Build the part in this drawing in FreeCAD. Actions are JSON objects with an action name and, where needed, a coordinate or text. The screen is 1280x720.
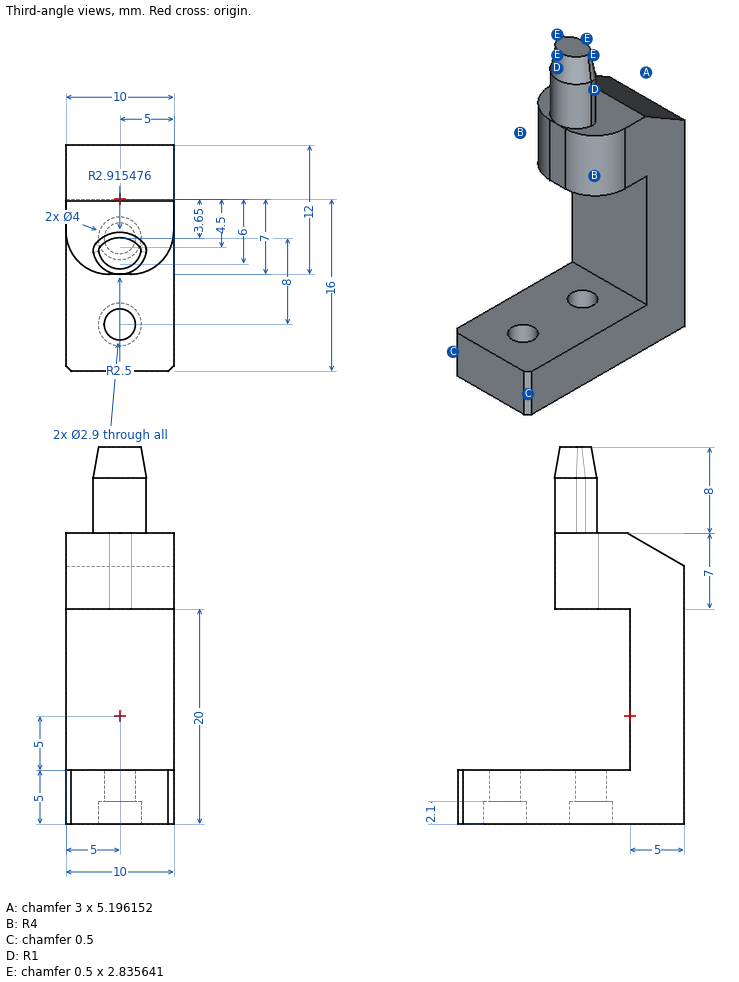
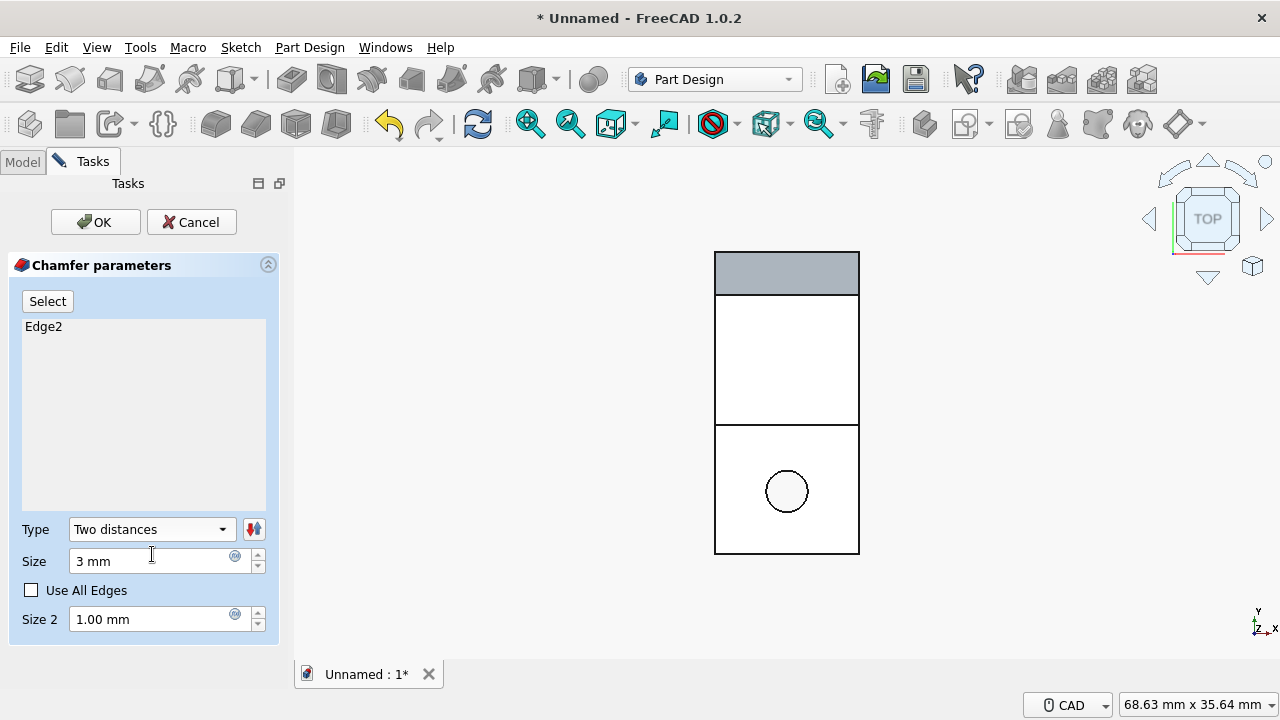
{"action": "triple_click", "coordinate": [160, 619]}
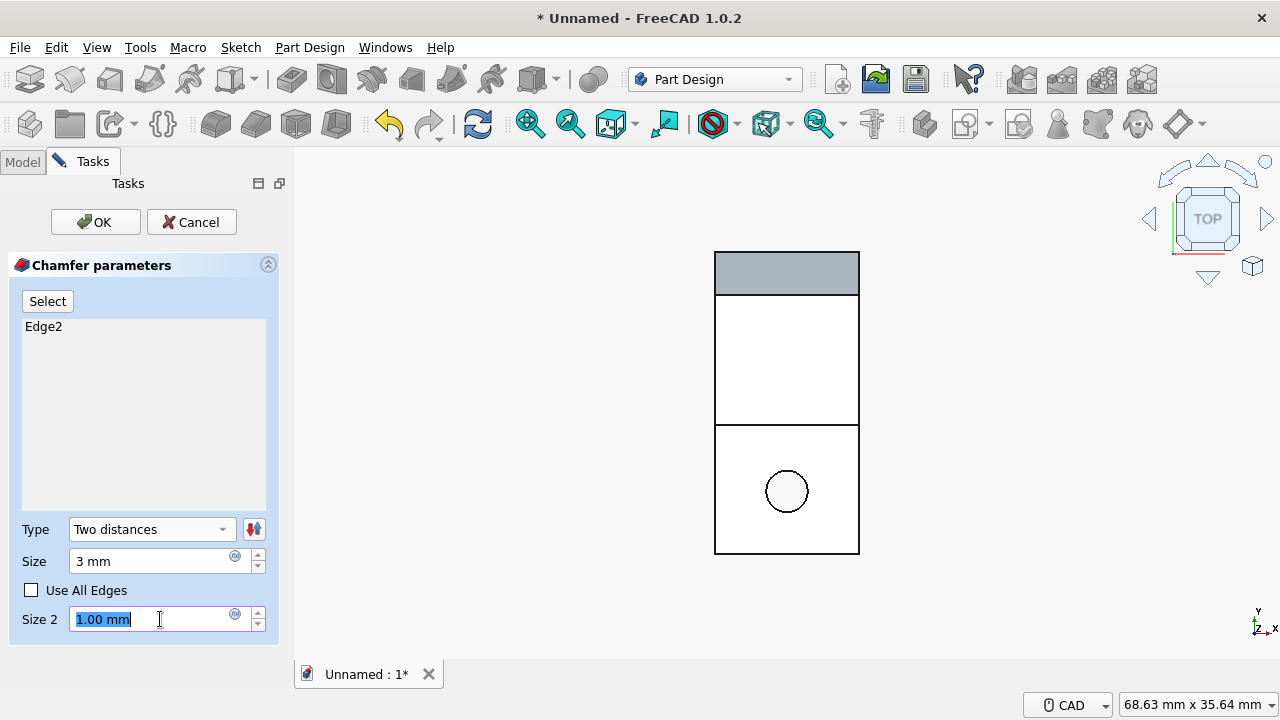
{"action": "type", "text": "5.196152"}
{"action": "key", "text": "Tab"}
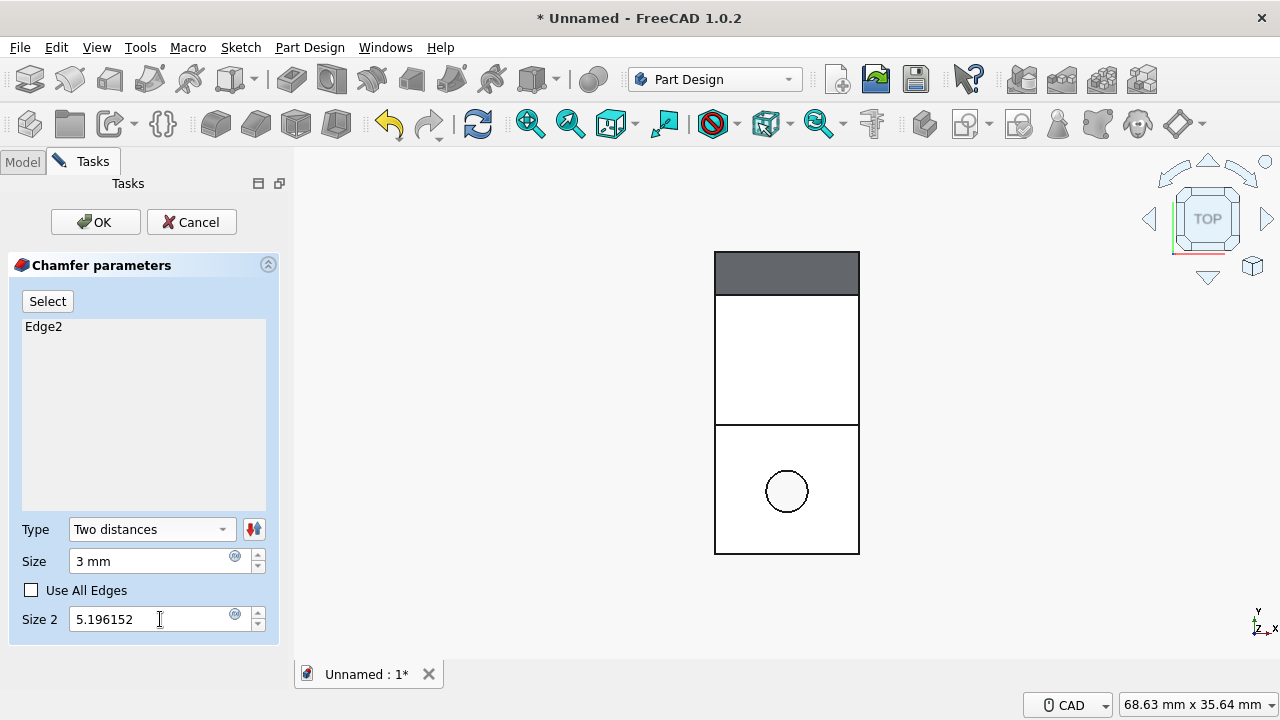
{"action": "left_click", "coordinate": [254, 530]}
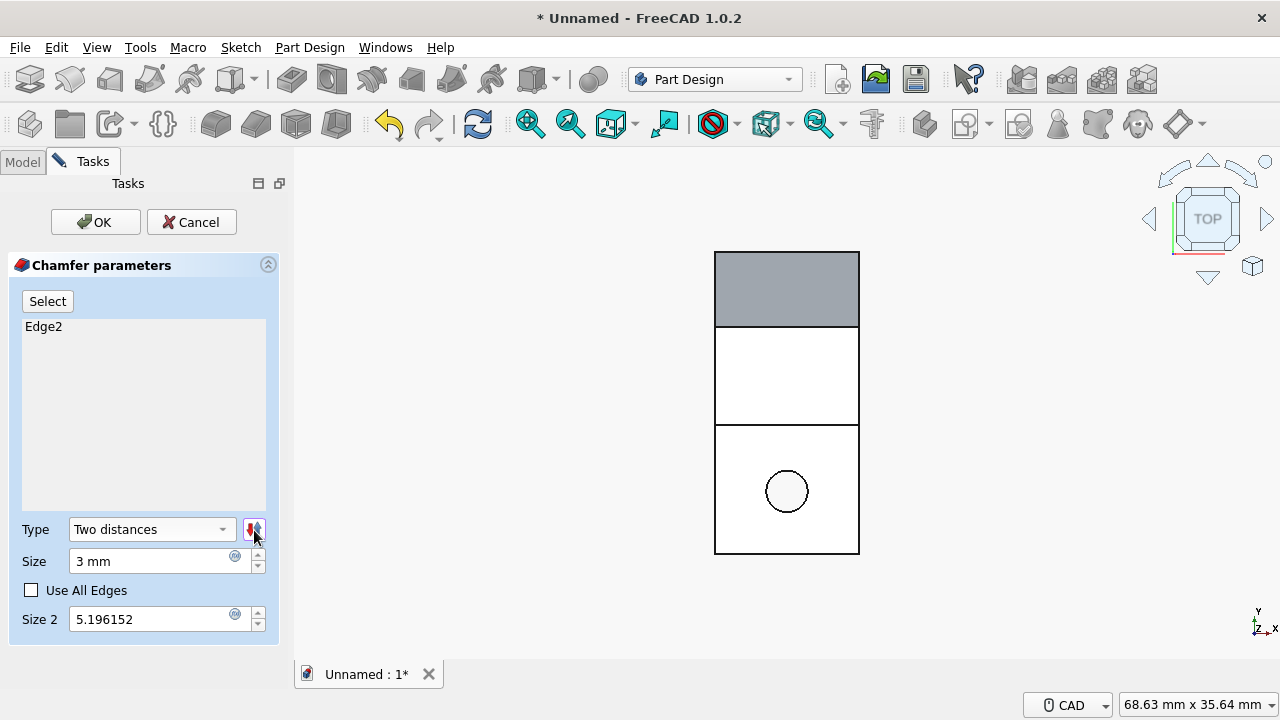
{"action": "left_click", "coordinate": [96, 222]}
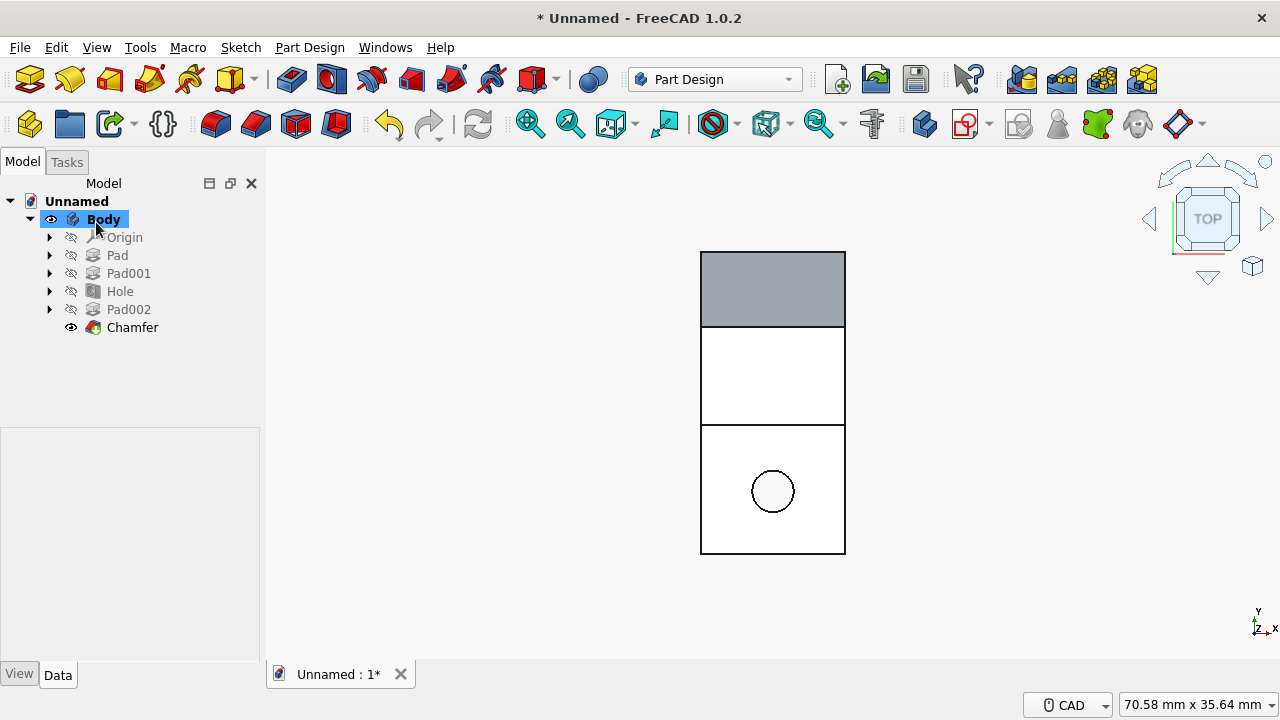
{"action": "key", "text": "0"}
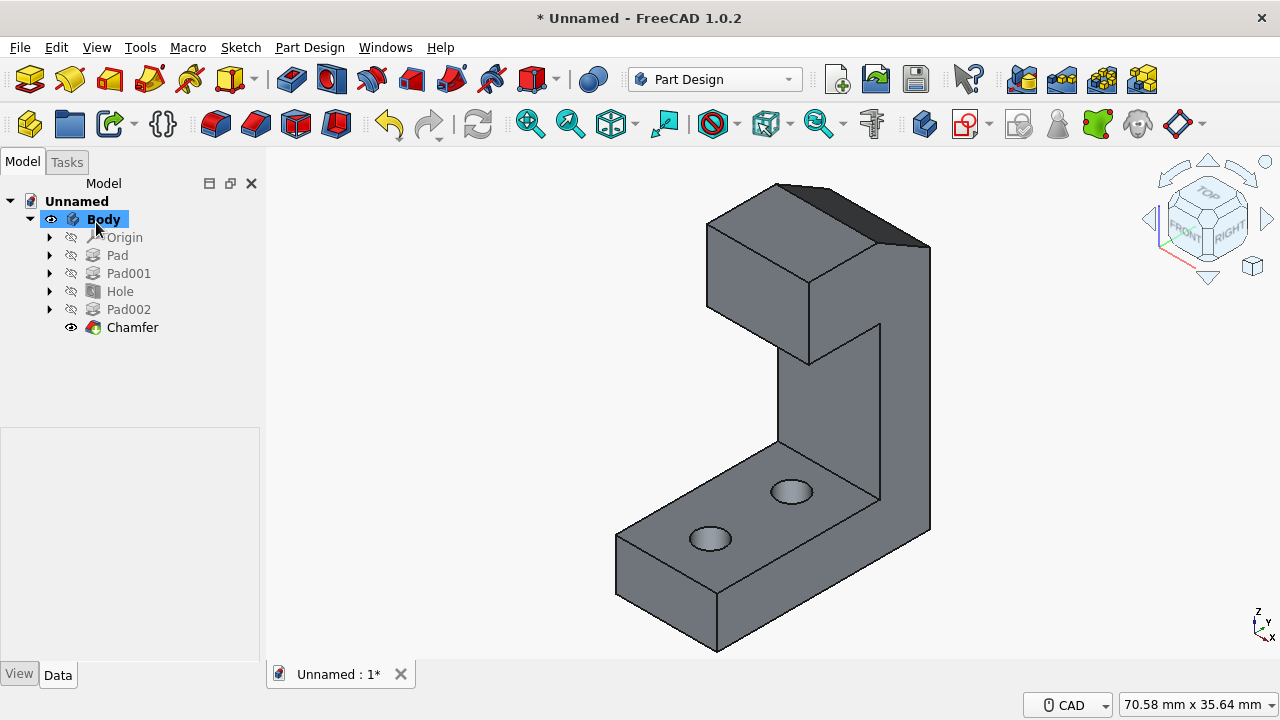
{"action": "left_click", "coordinate": [809, 323]}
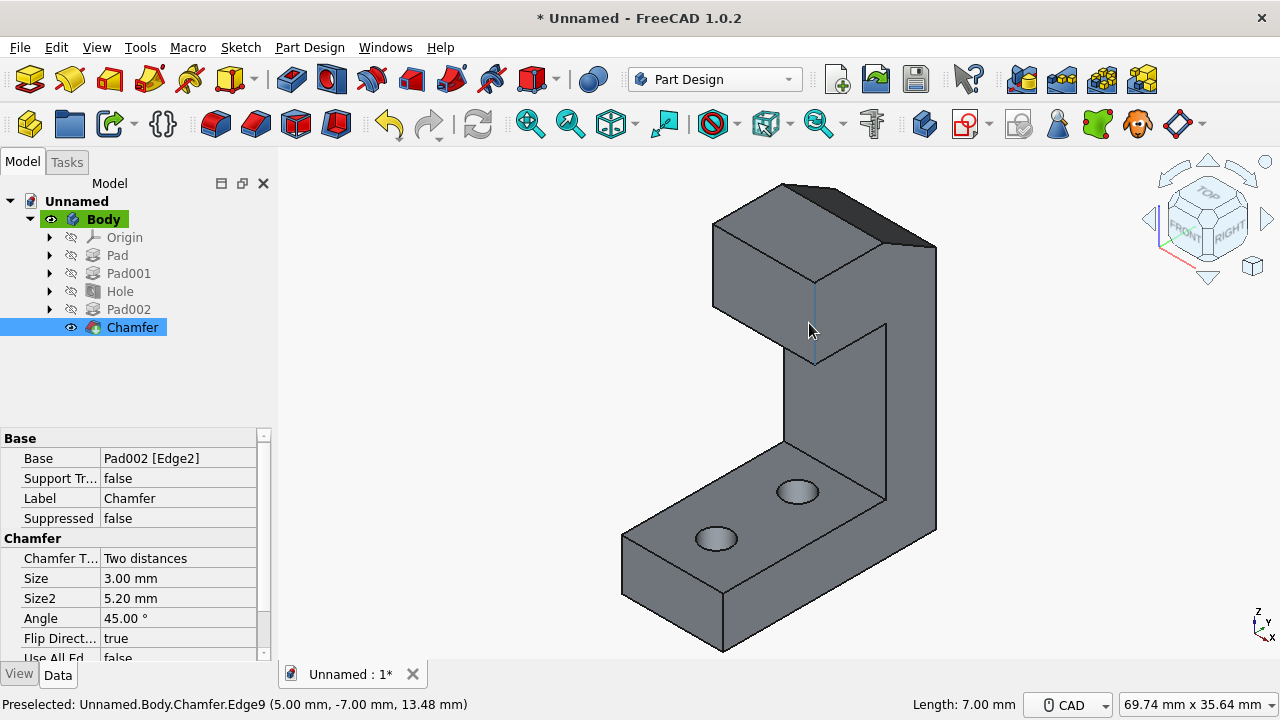
{"action": "key", "text": "2"}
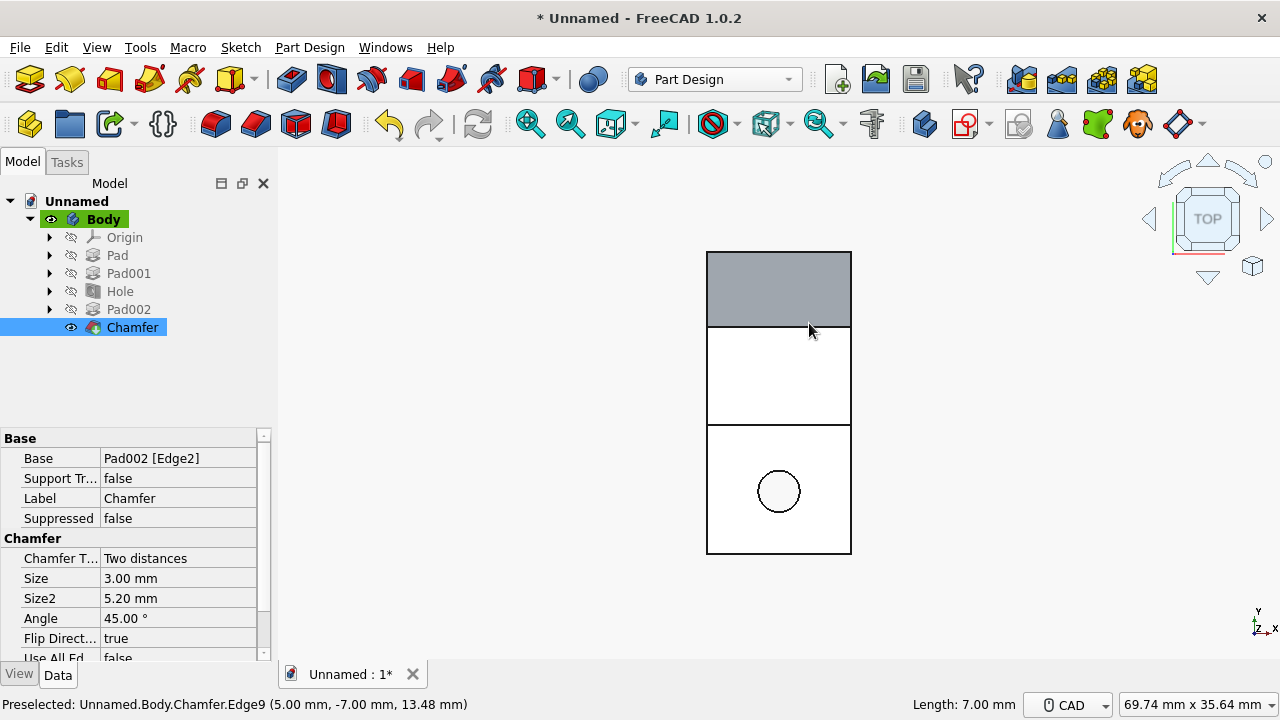
{"action": "key", "text": "1"}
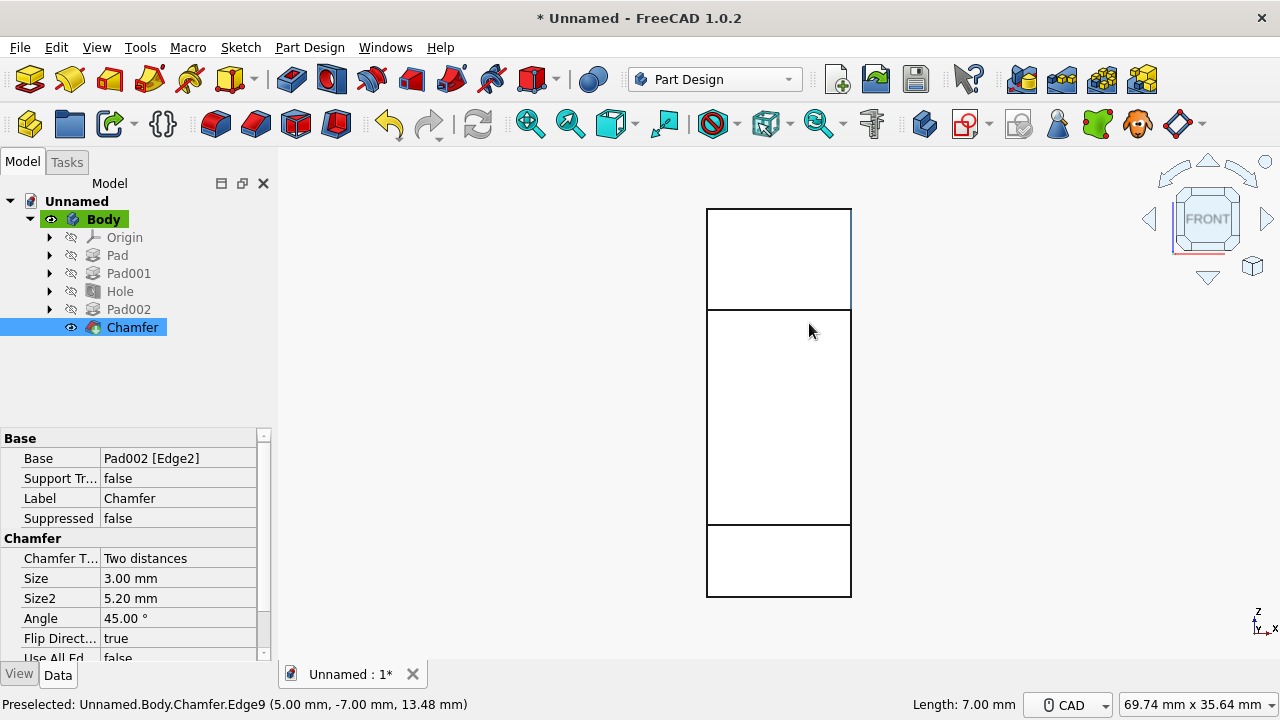
{"action": "left_click", "coordinate": [707, 258], "text": "ctrl"}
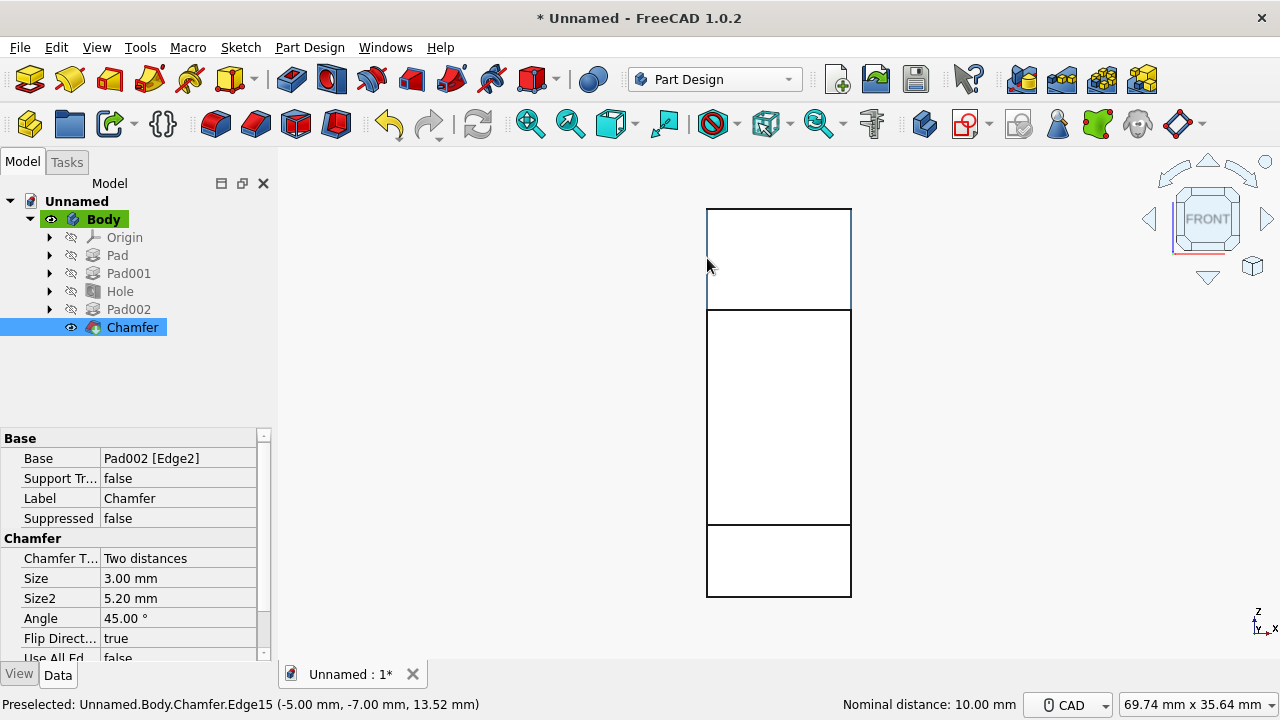
{"action": "left_click", "coordinate": [216, 124]}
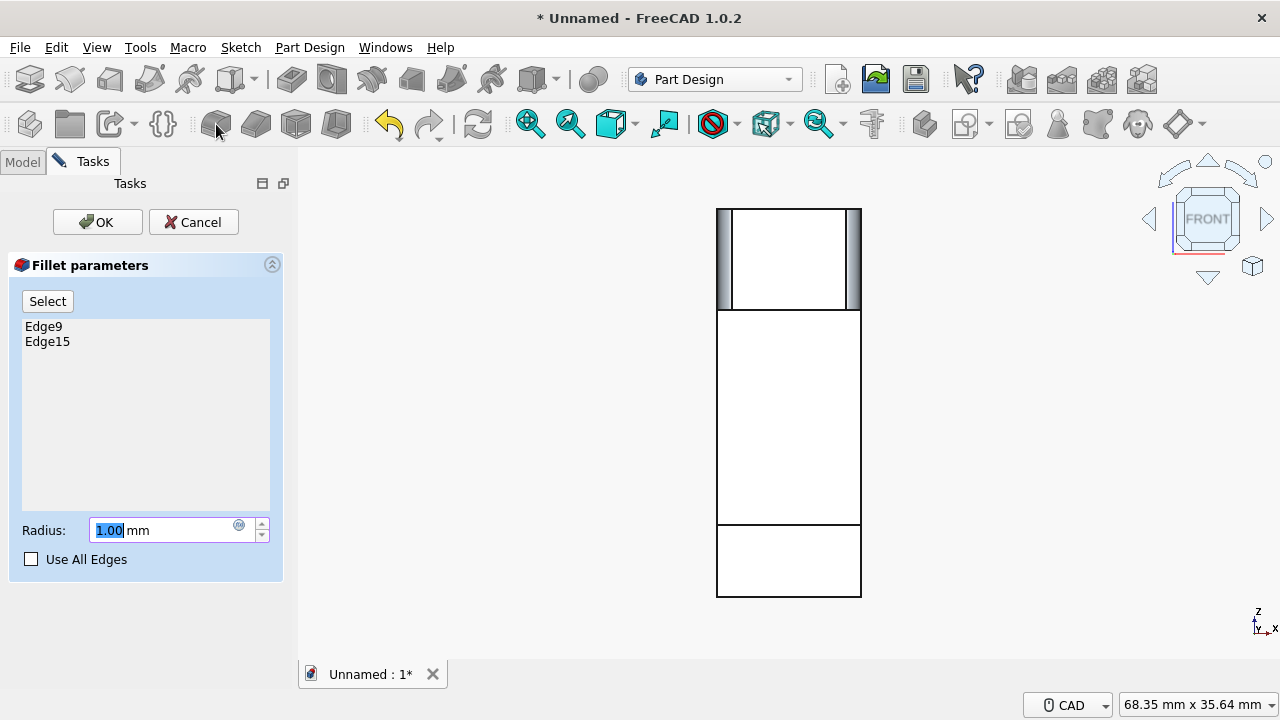
{"action": "type", "text": "4"}
{"action": "key", "text": "Tab"}